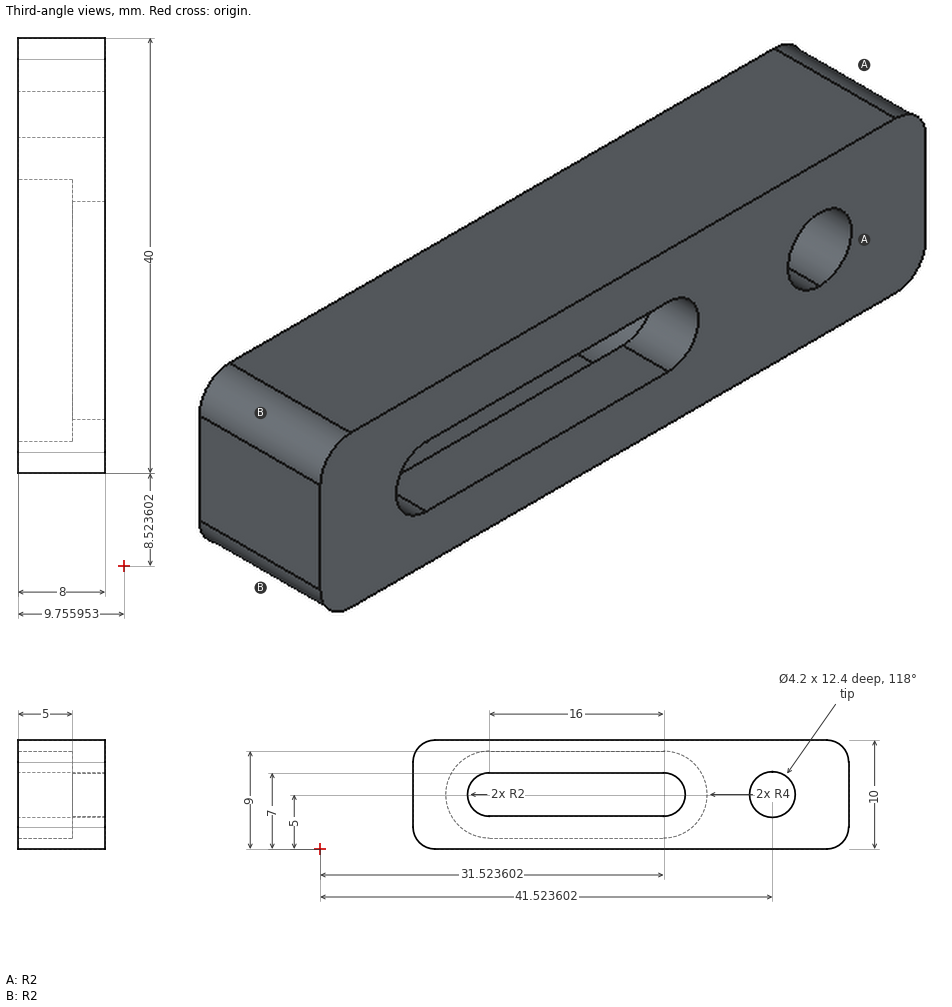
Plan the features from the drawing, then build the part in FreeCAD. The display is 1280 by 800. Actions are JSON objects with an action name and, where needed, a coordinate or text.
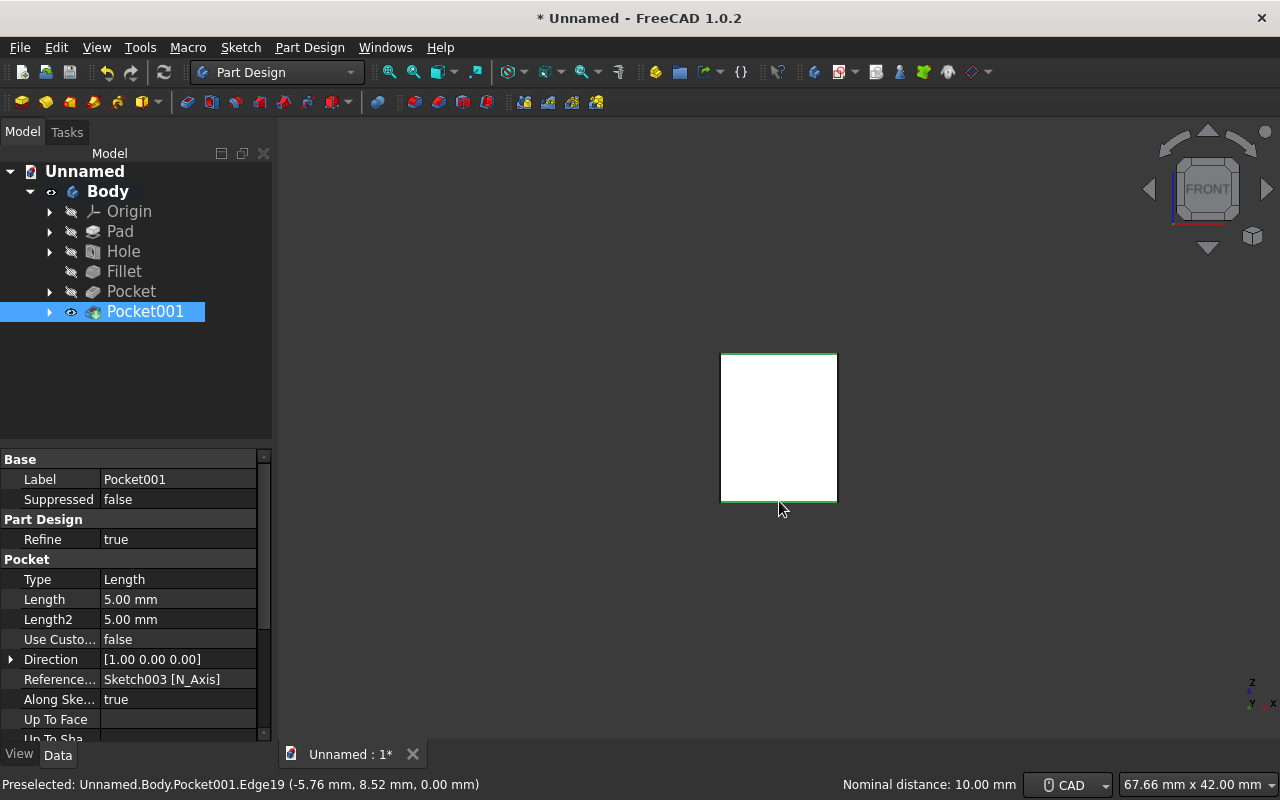
{"action": "left_click", "coordinate": [416, 102]}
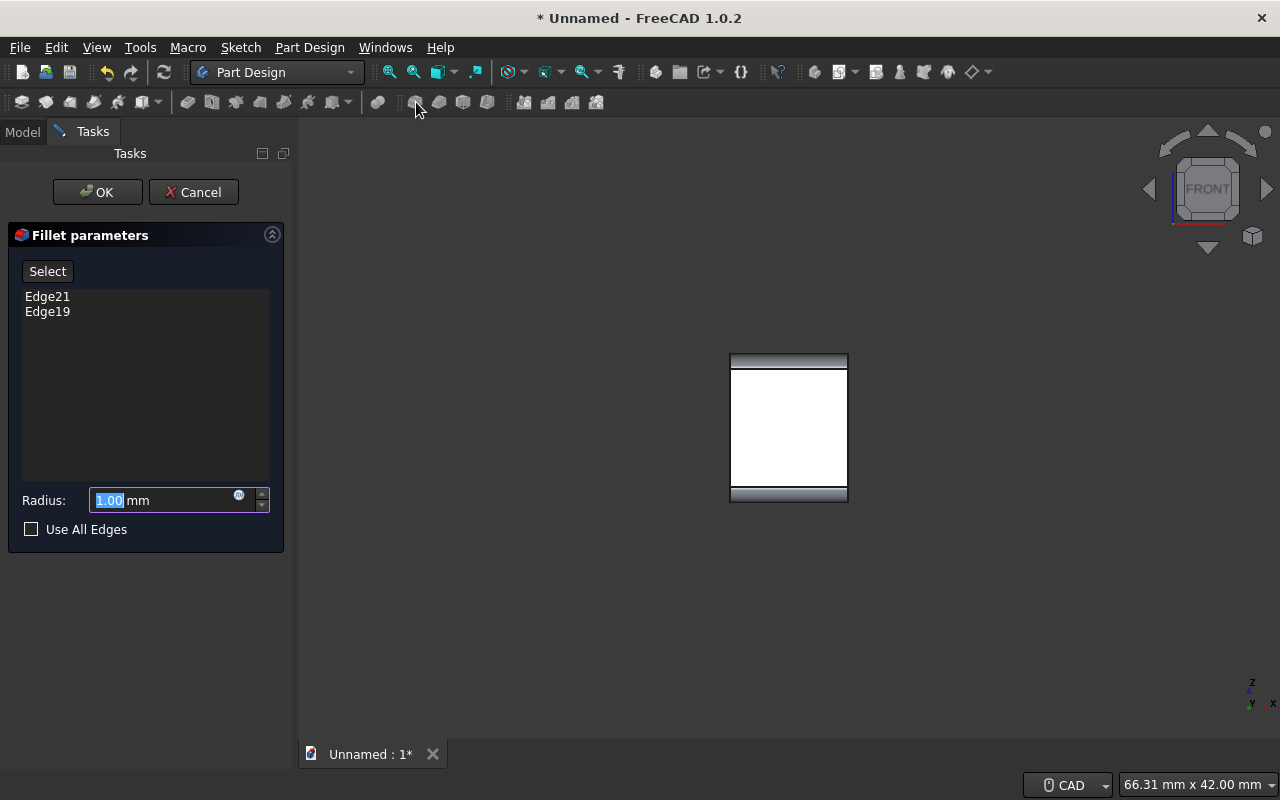
{"action": "type", "text": "2"}
{"action": "key", "text": "Tab"}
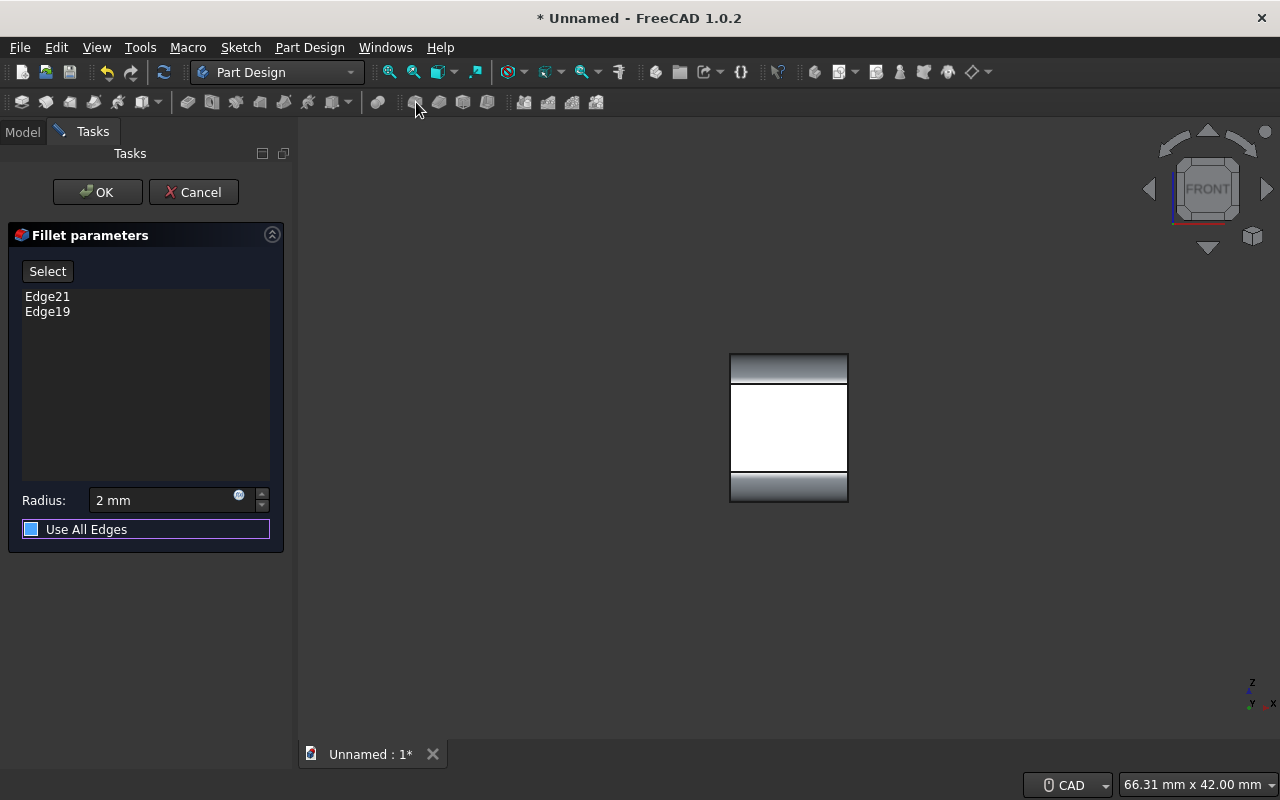
{"action": "left_click", "coordinate": [98, 192]}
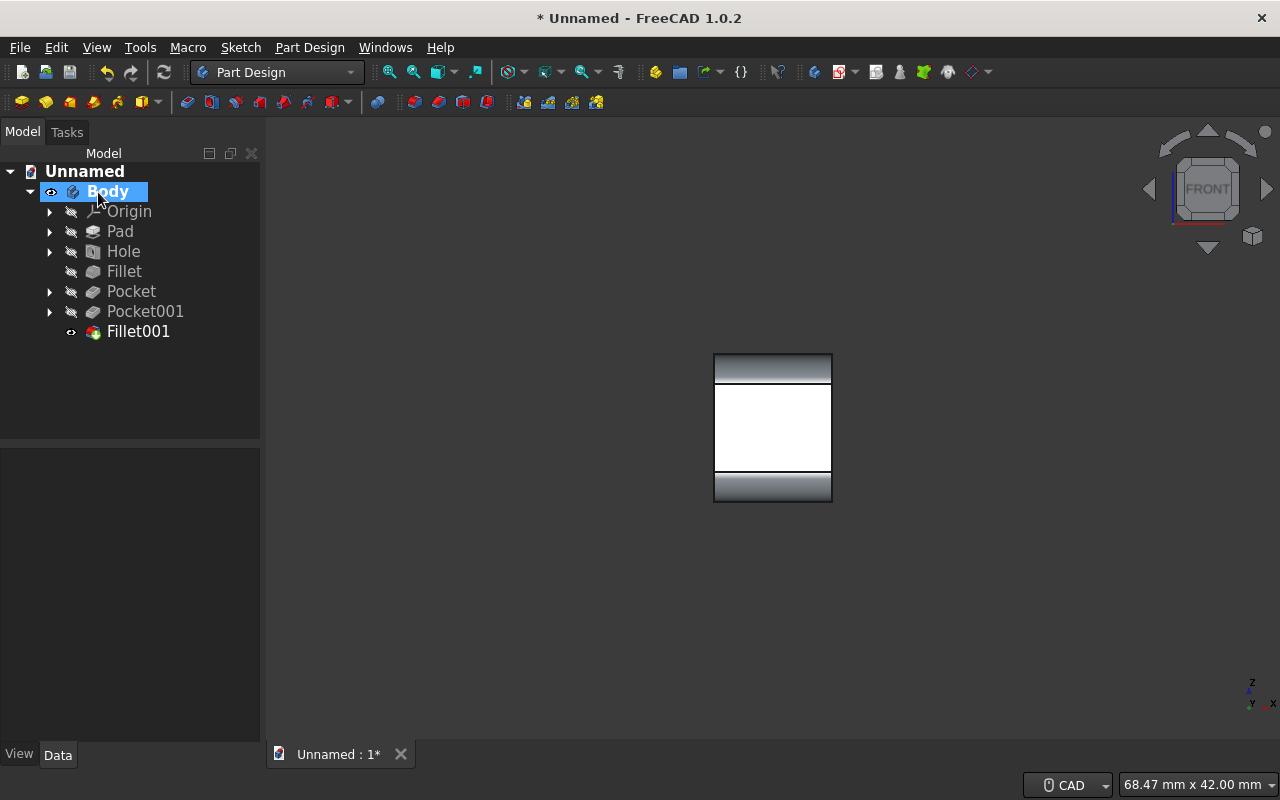
{"action": "key", "text": "0"}